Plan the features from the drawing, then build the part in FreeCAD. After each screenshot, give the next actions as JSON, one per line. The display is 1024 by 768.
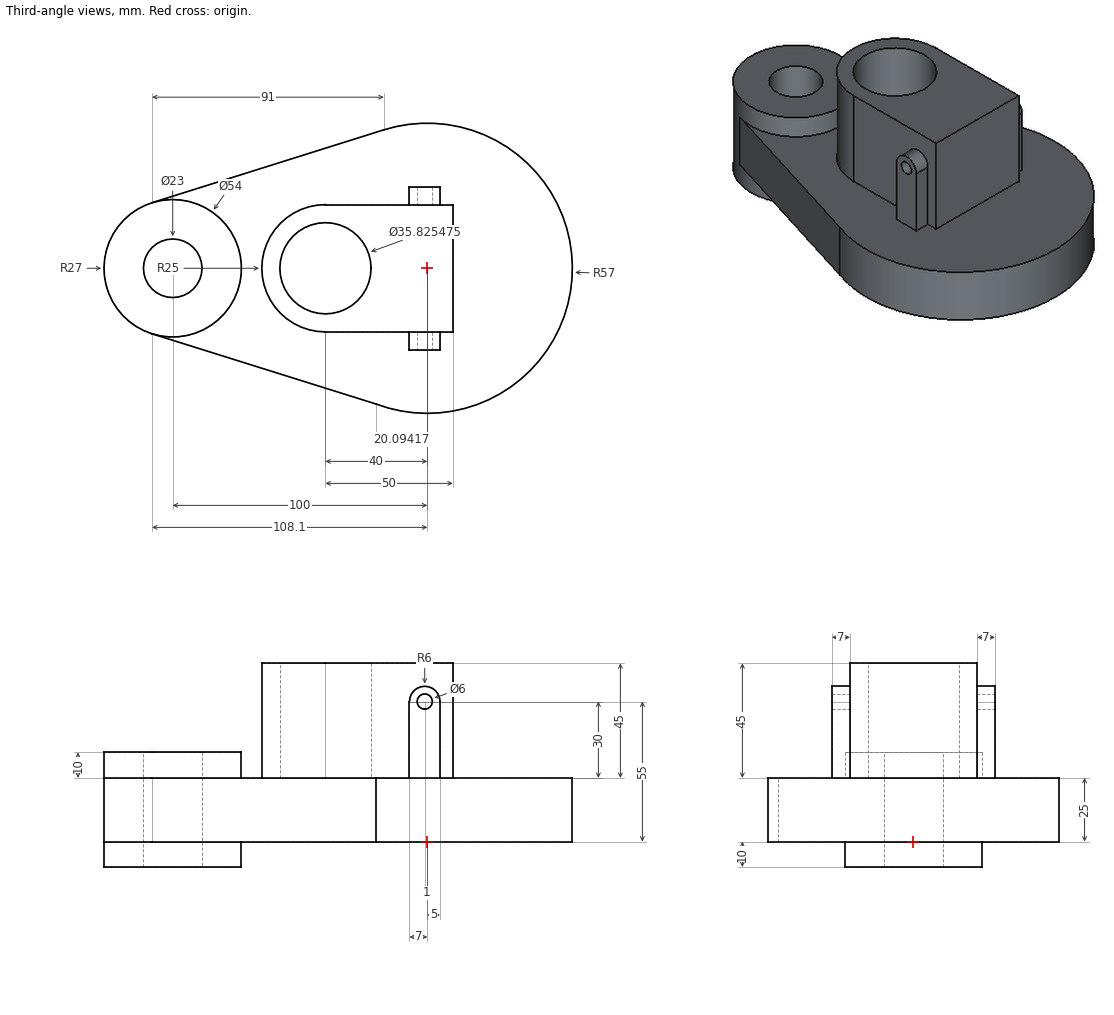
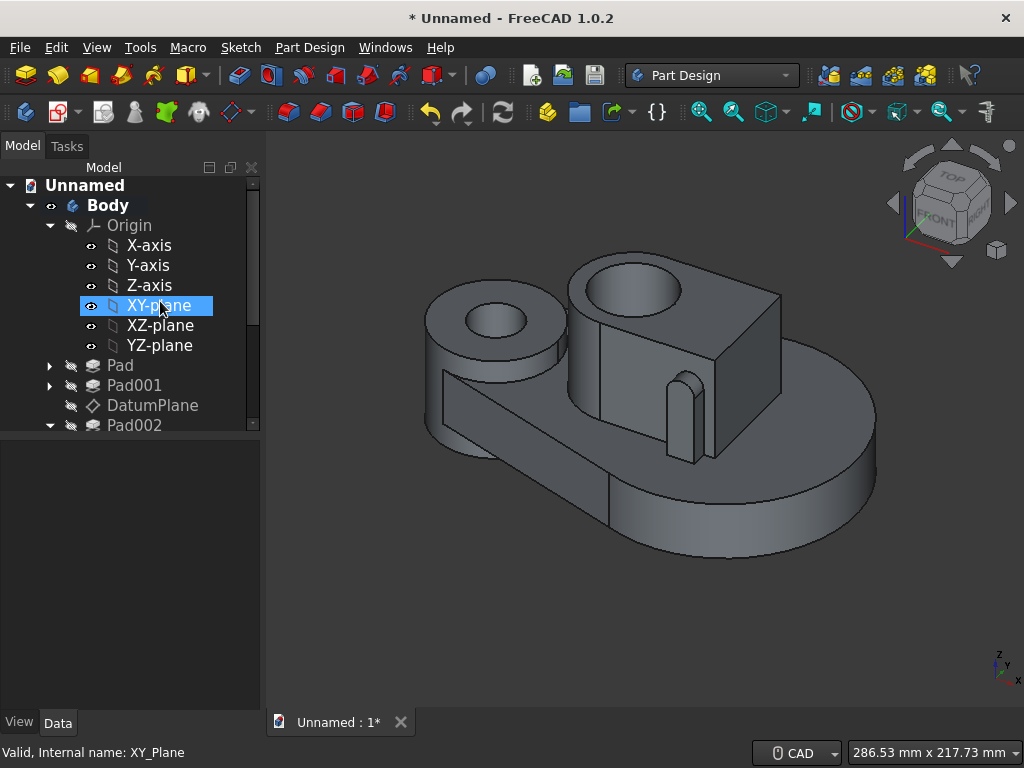
{"action": "left_click", "coordinate": [136, 326]}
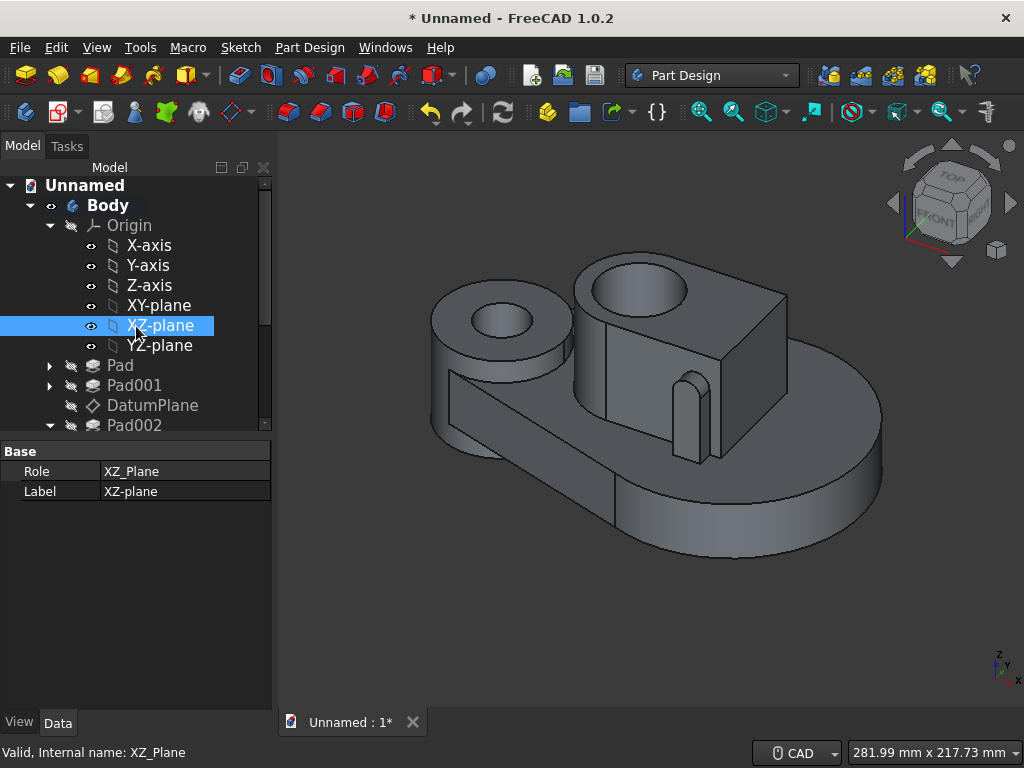
{"action": "left_click", "coordinate": [232, 112]}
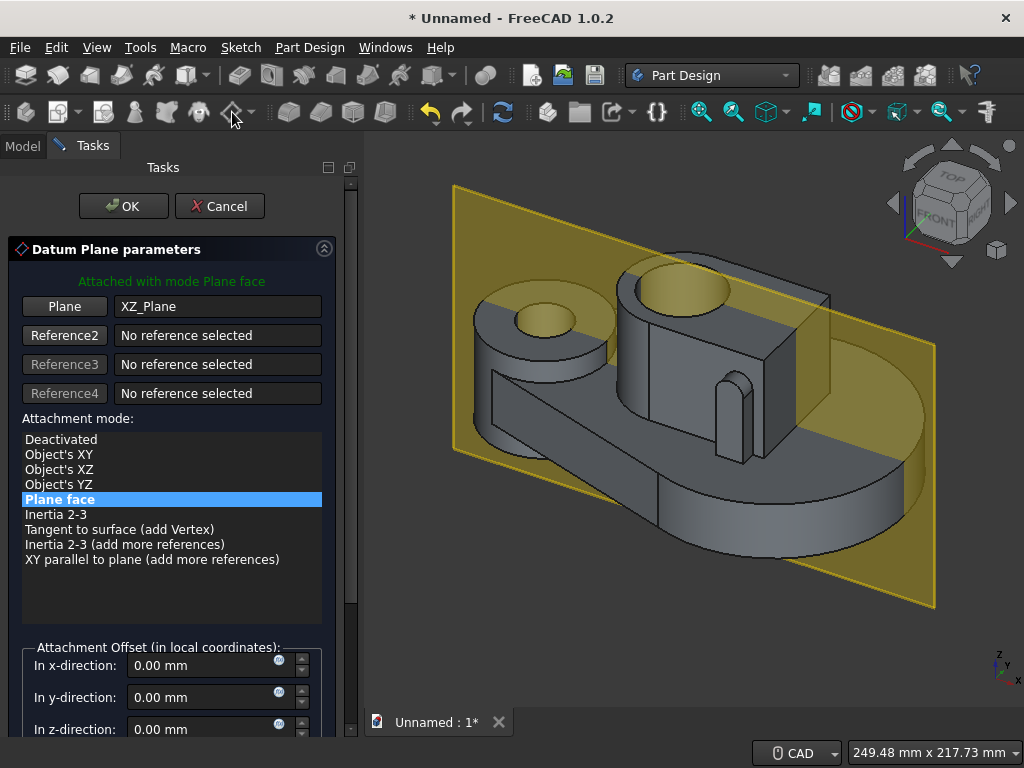
{"action": "scroll", "coordinate": [351, 456], "scroll_direction": "down", "scroll_amount": 2}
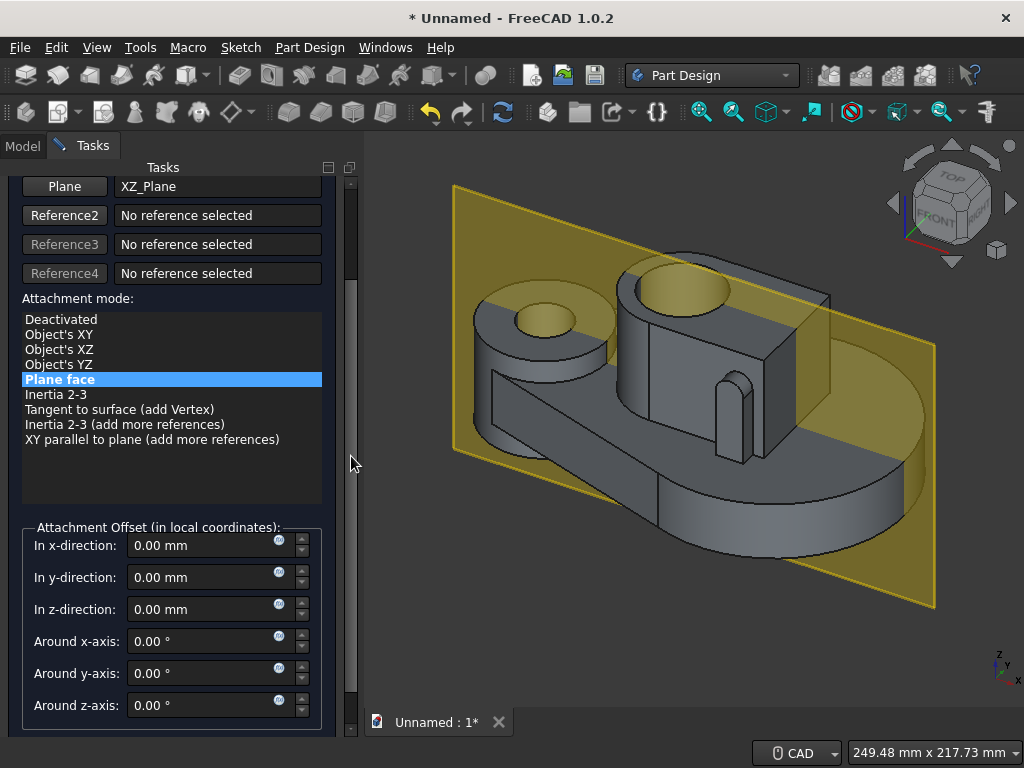
{"action": "triple_click", "coordinate": [210, 609]}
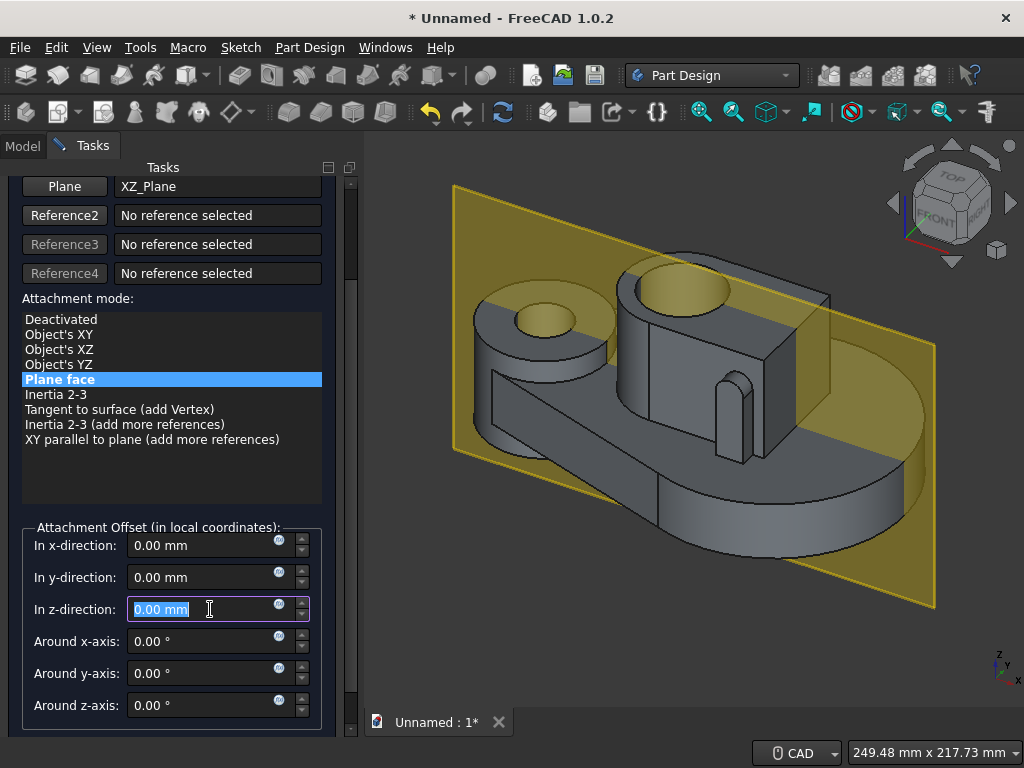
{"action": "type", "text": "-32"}
{"action": "key", "text": "Tab"}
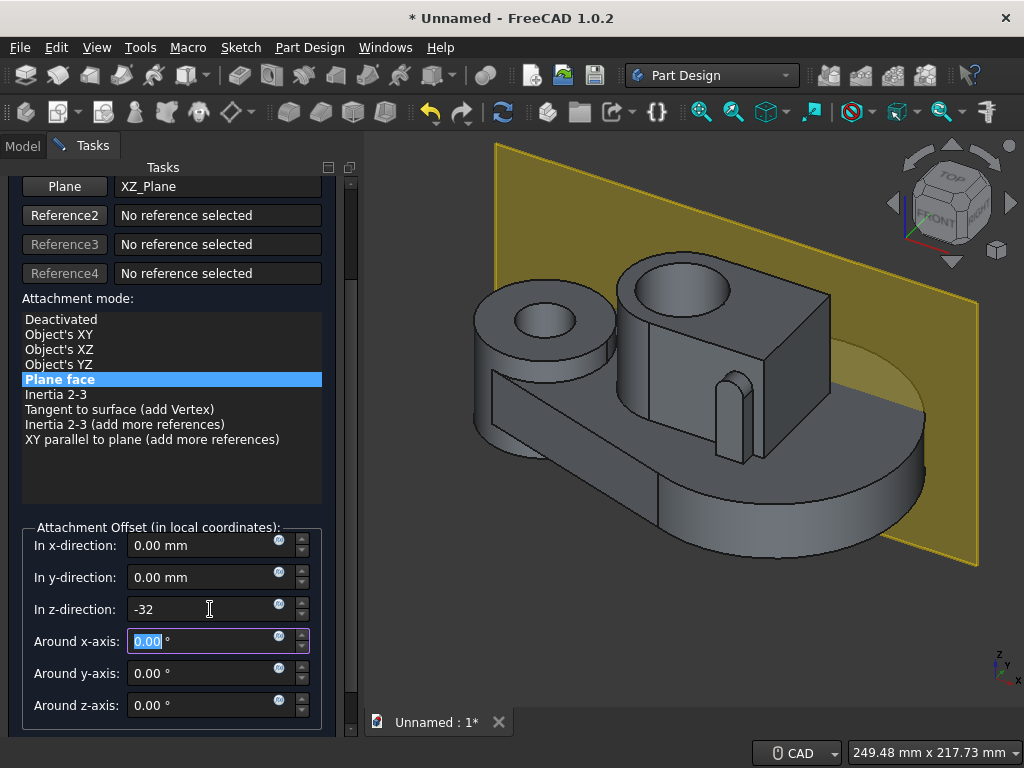
{"action": "scroll", "coordinate": [351, 456], "scroll_direction": "up", "scroll_amount": 3}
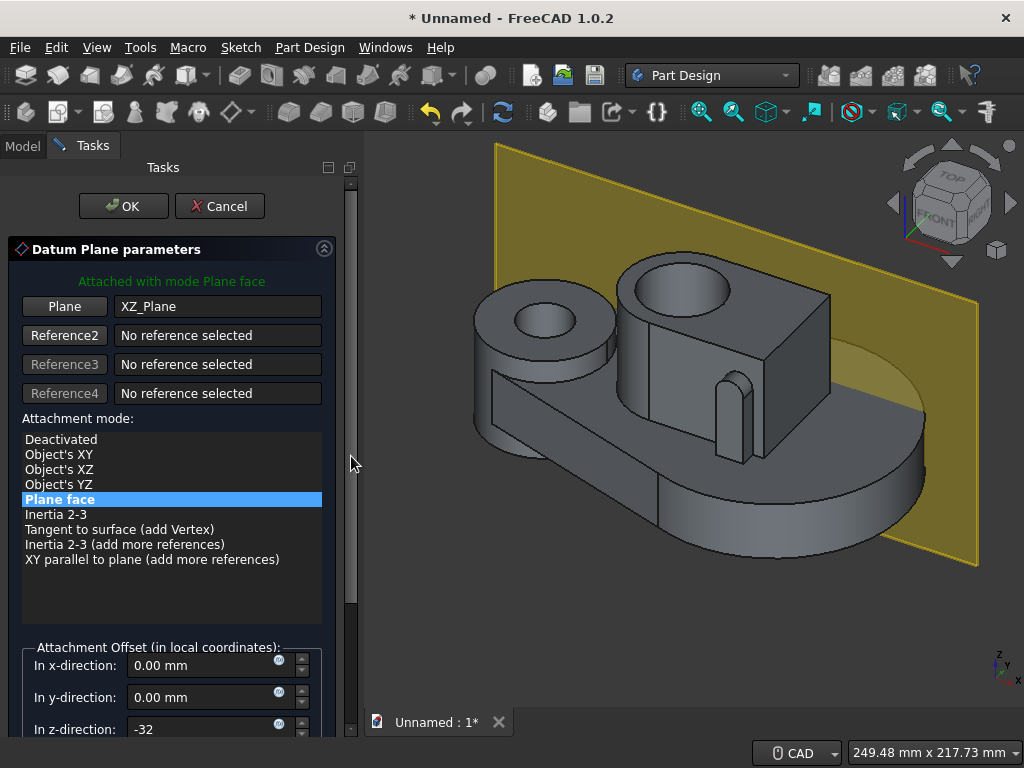
{"action": "left_click", "coordinate": [124, 206]}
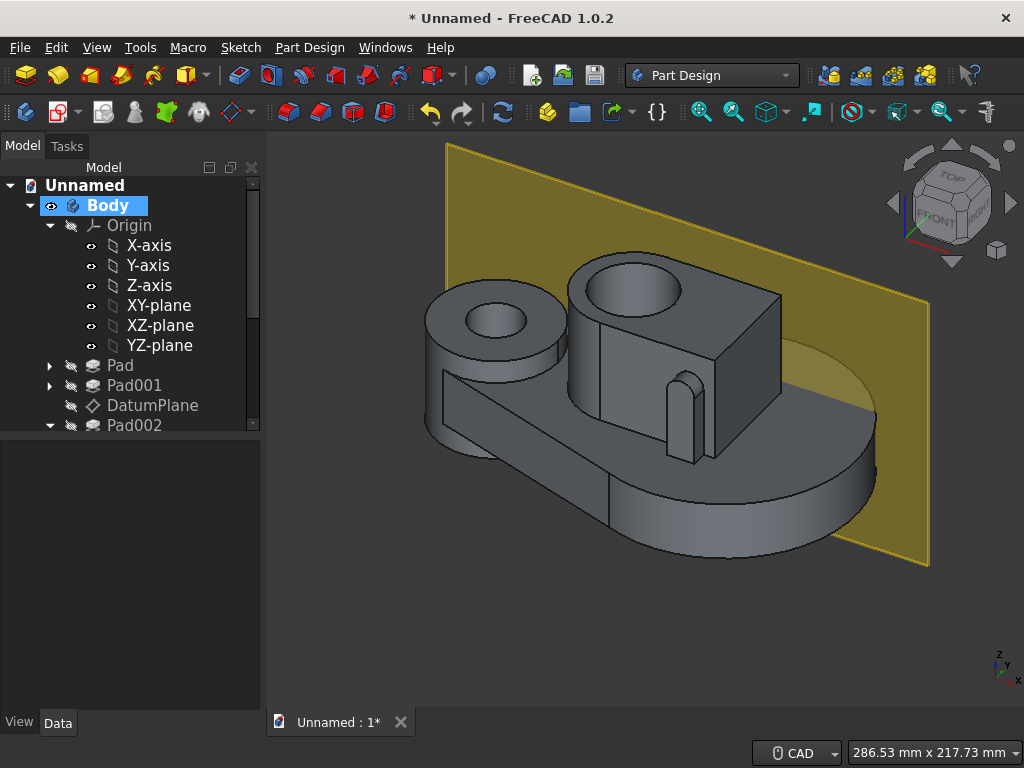
{"action": "scroll", "coordinate": [100, 301], "scroll_direction": "down", "scroll_amount": 3}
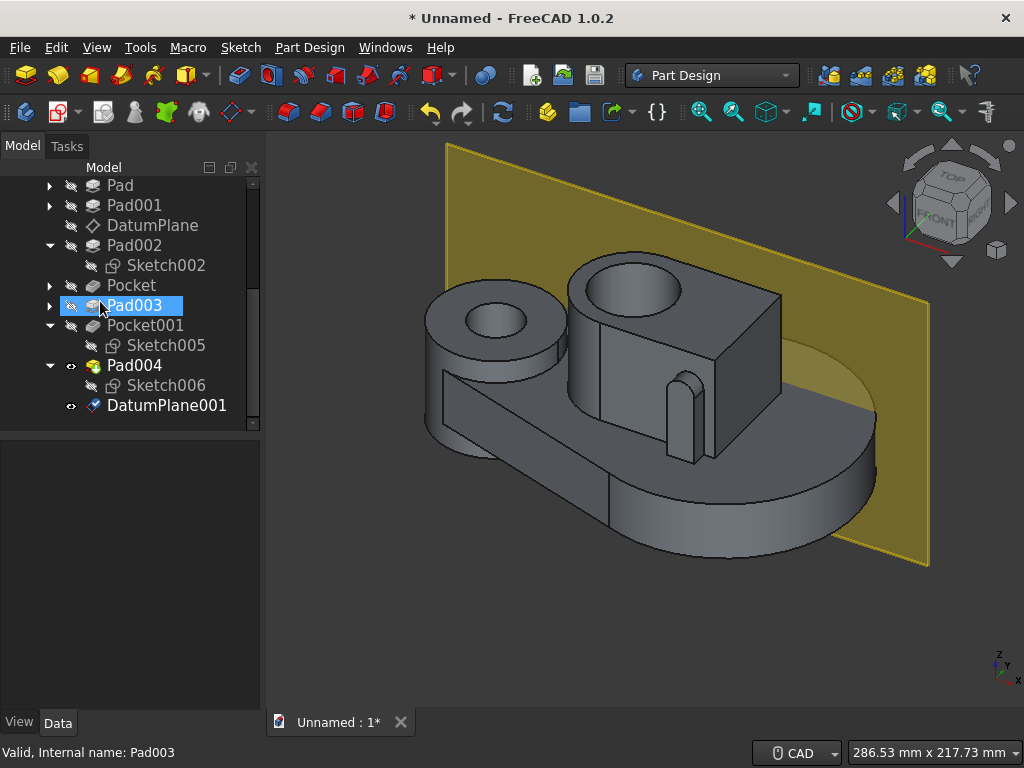
{"action": "left_click", "coordinate": [116, 406]}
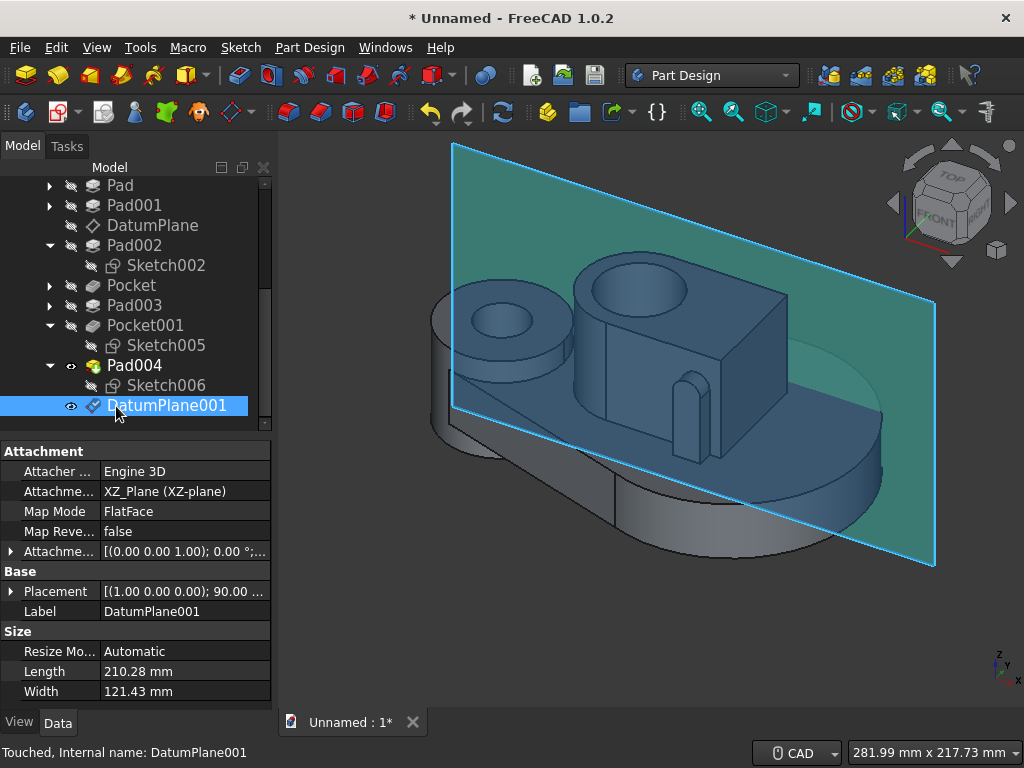
{"action": "left_click", "coordinate": [58, 112]}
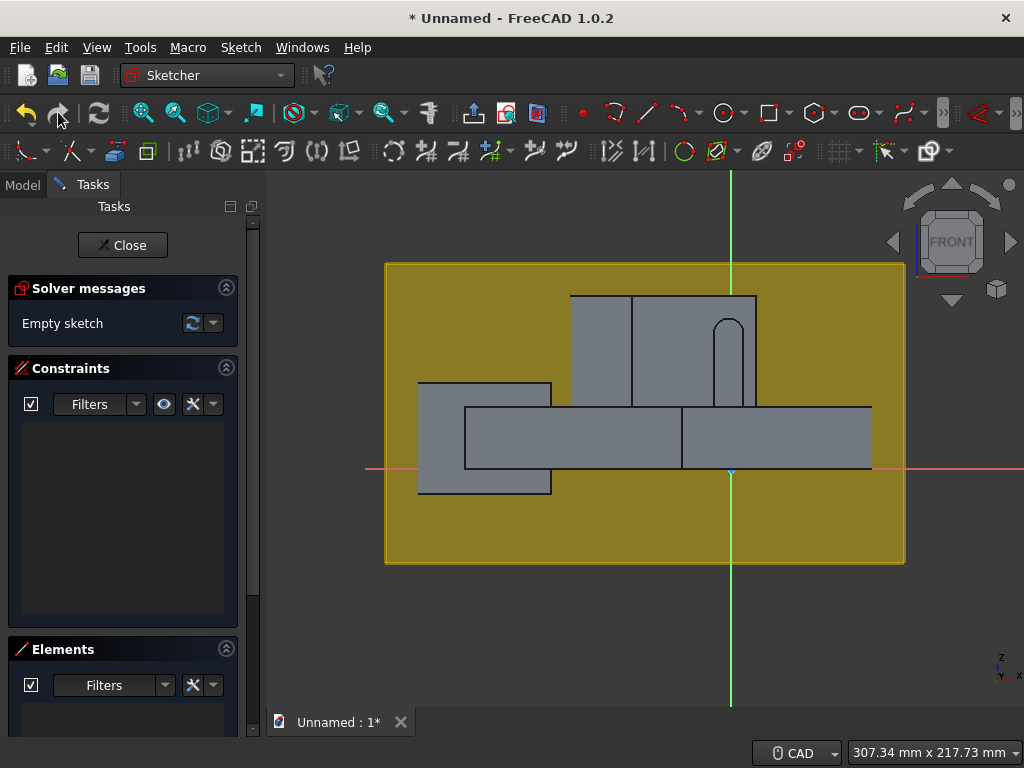
{"action": "key", "text": "q s"}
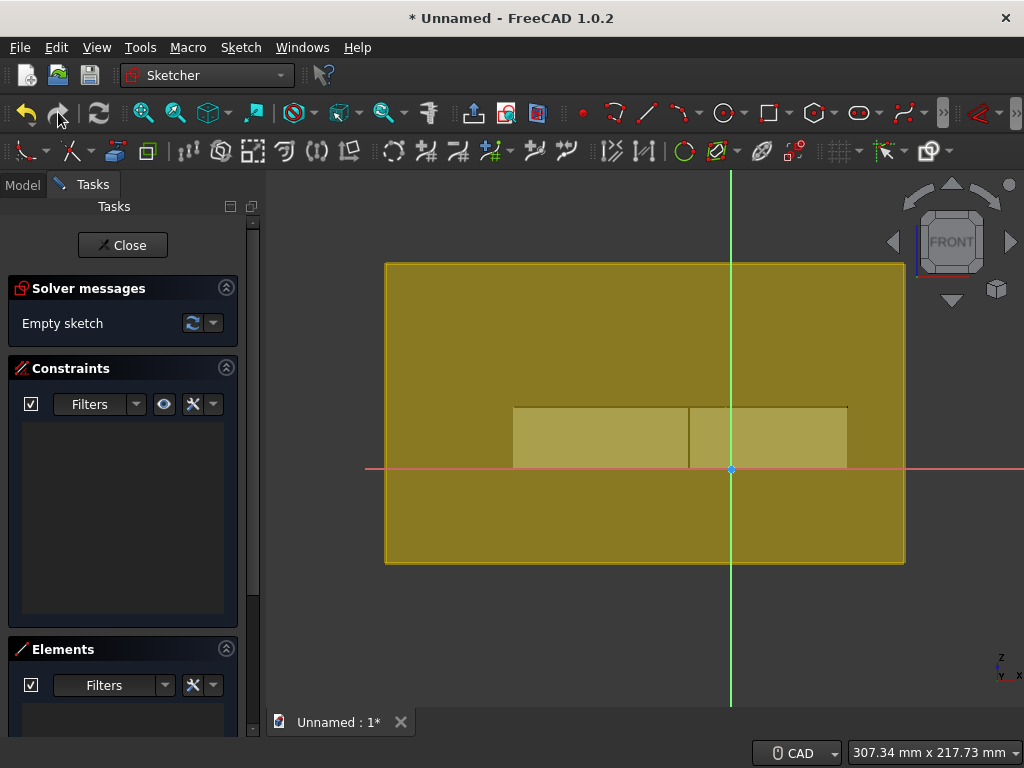
{"action": "scroll", "coordinate": [853, 357], "scroll_direction": "up", "scroll_amount": 4}